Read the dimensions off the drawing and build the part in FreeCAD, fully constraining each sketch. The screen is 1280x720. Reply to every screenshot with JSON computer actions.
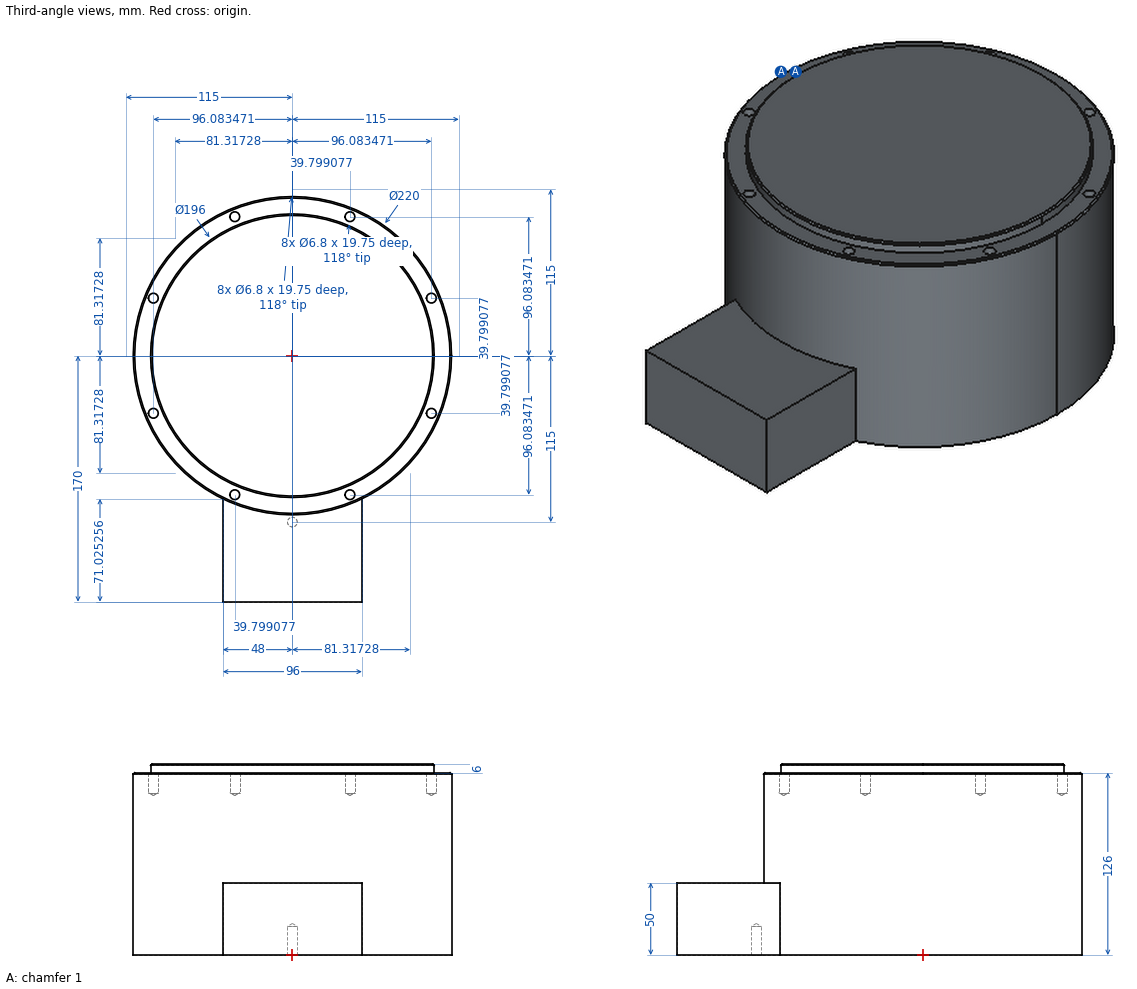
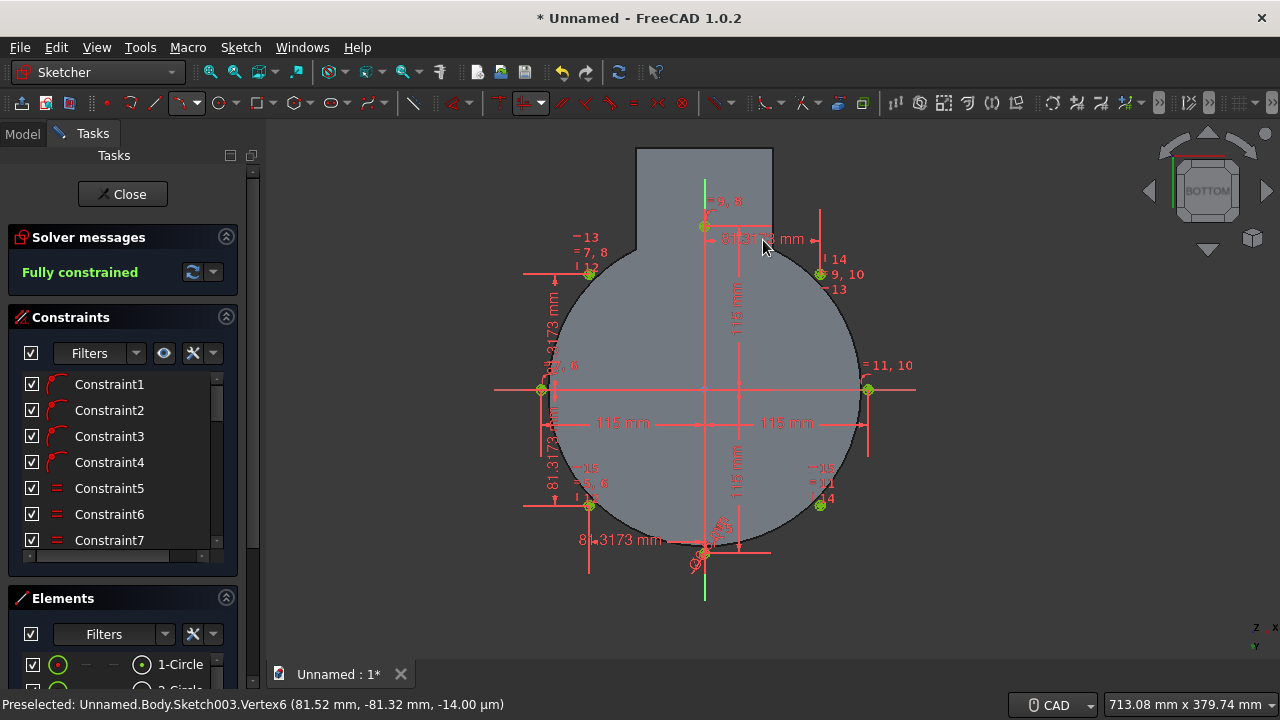
{"action": "left_click", "coordinate": [123, 194]}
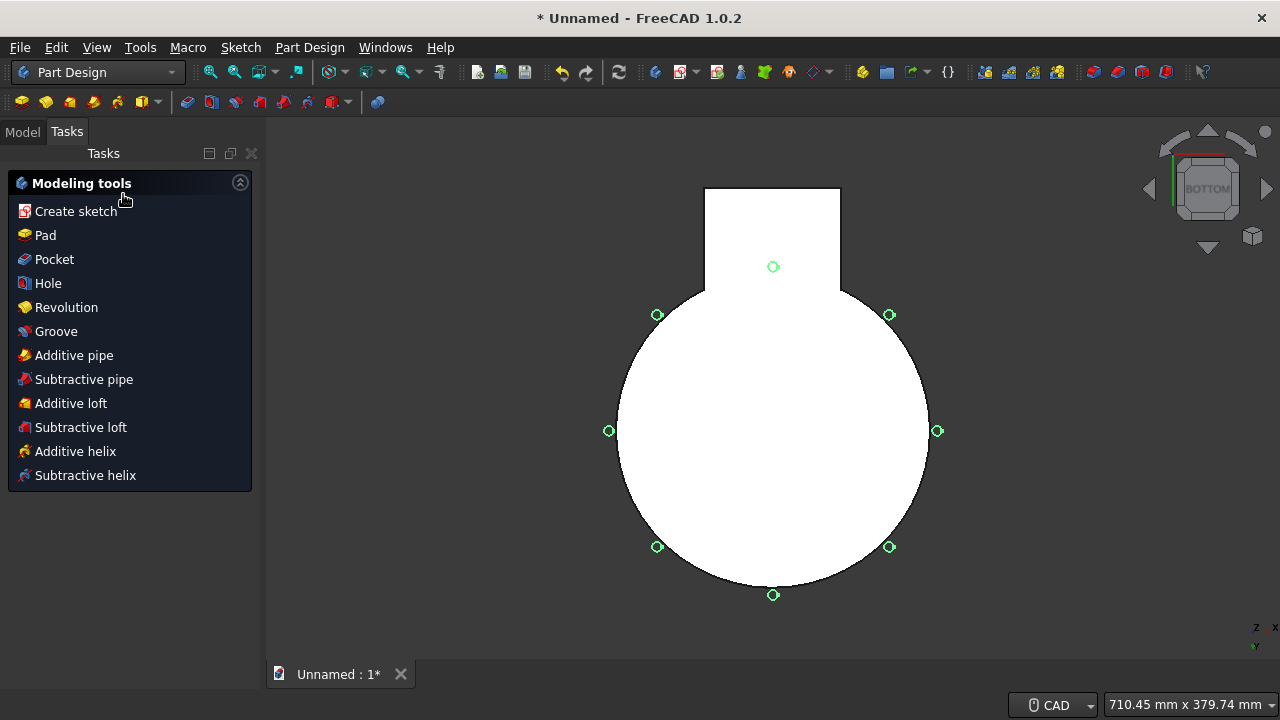
{"action": "left_click", "coordinate": [212, 102]}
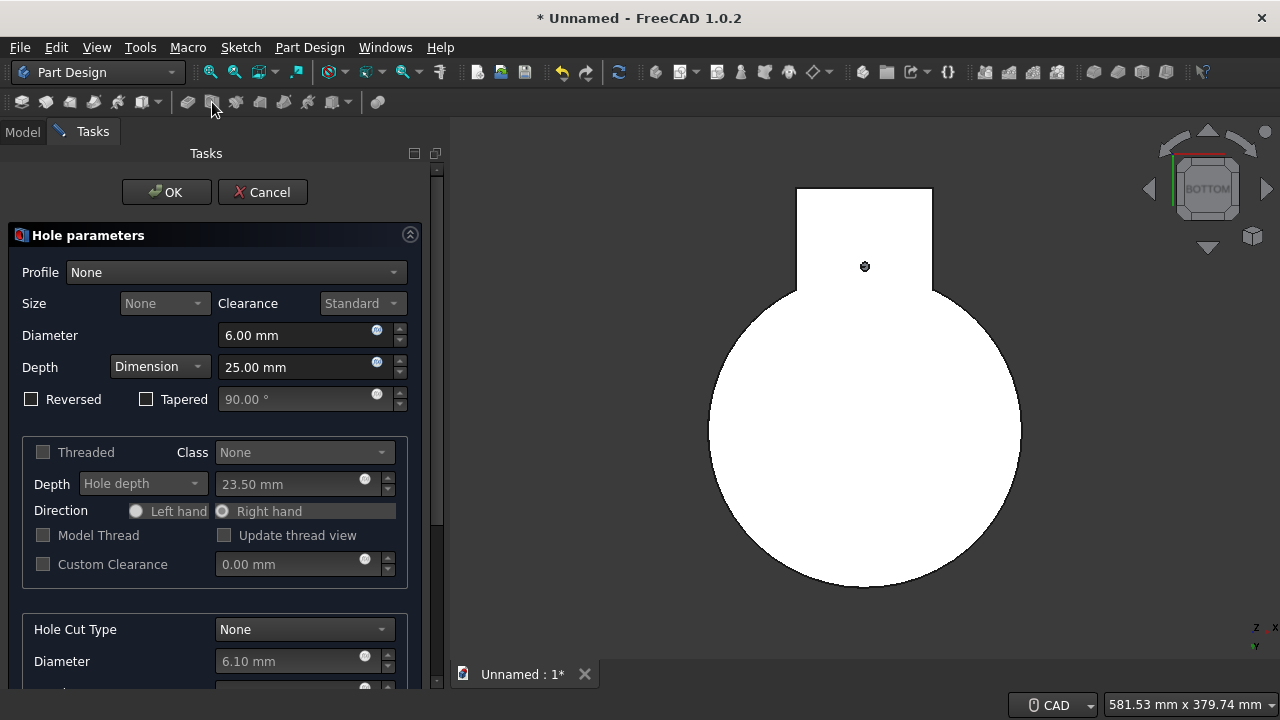
{"action": "triple_click", "coordinate": [305, 335]}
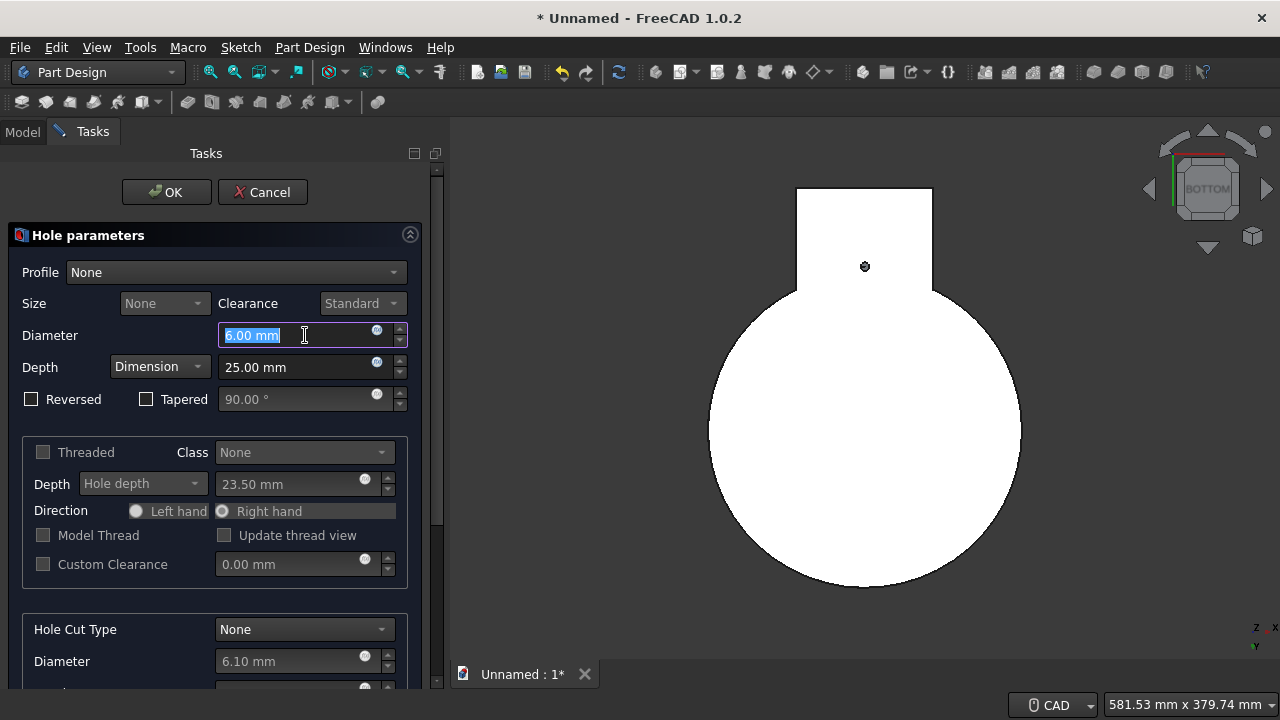
{"action": "type", "text": "6.8"}
{"action": "key", "text": "Tab"}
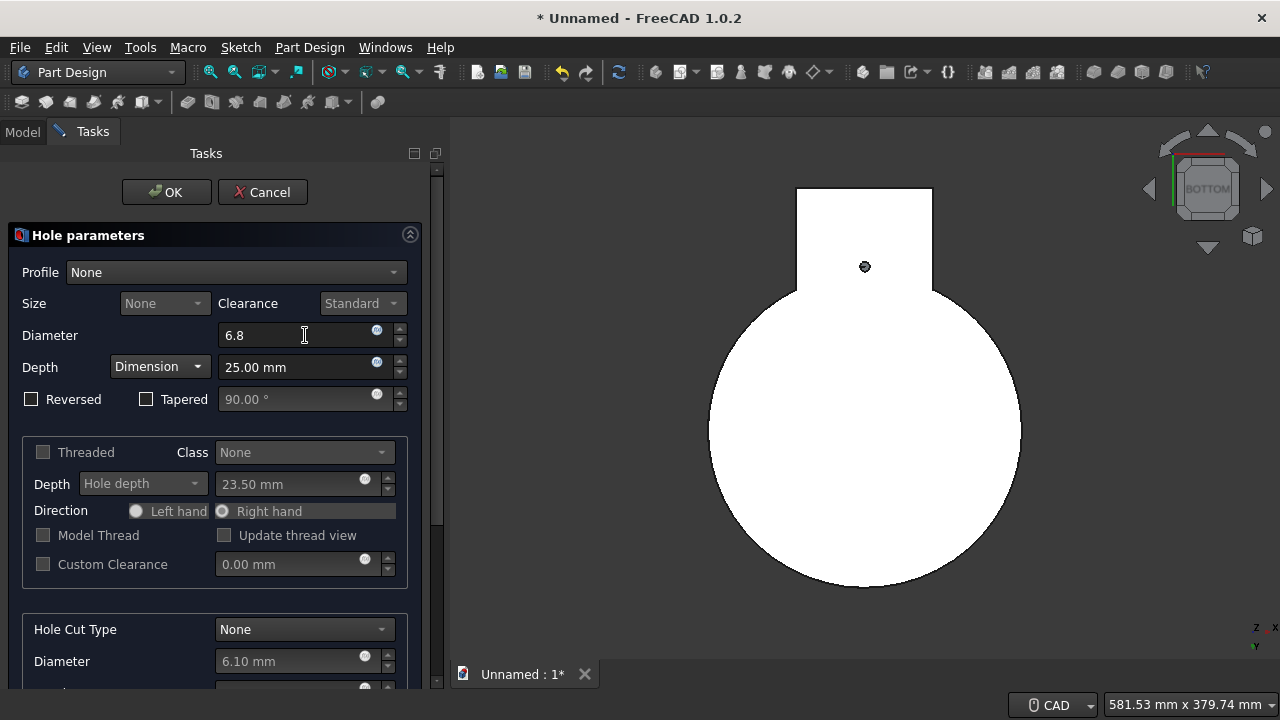
{"action": "triple_click", "coordinate": [305, 367]}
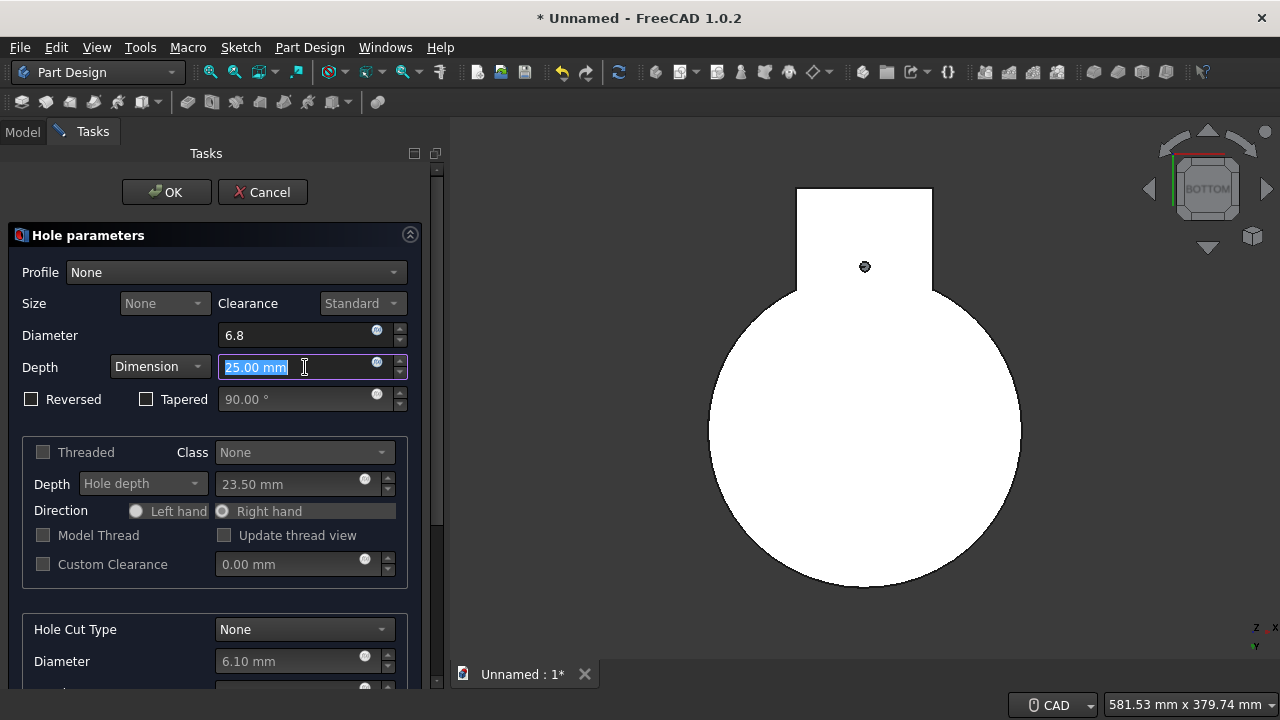
{"action": "type", "text": "19.75"}
{"action": "key", "text": "Tab"}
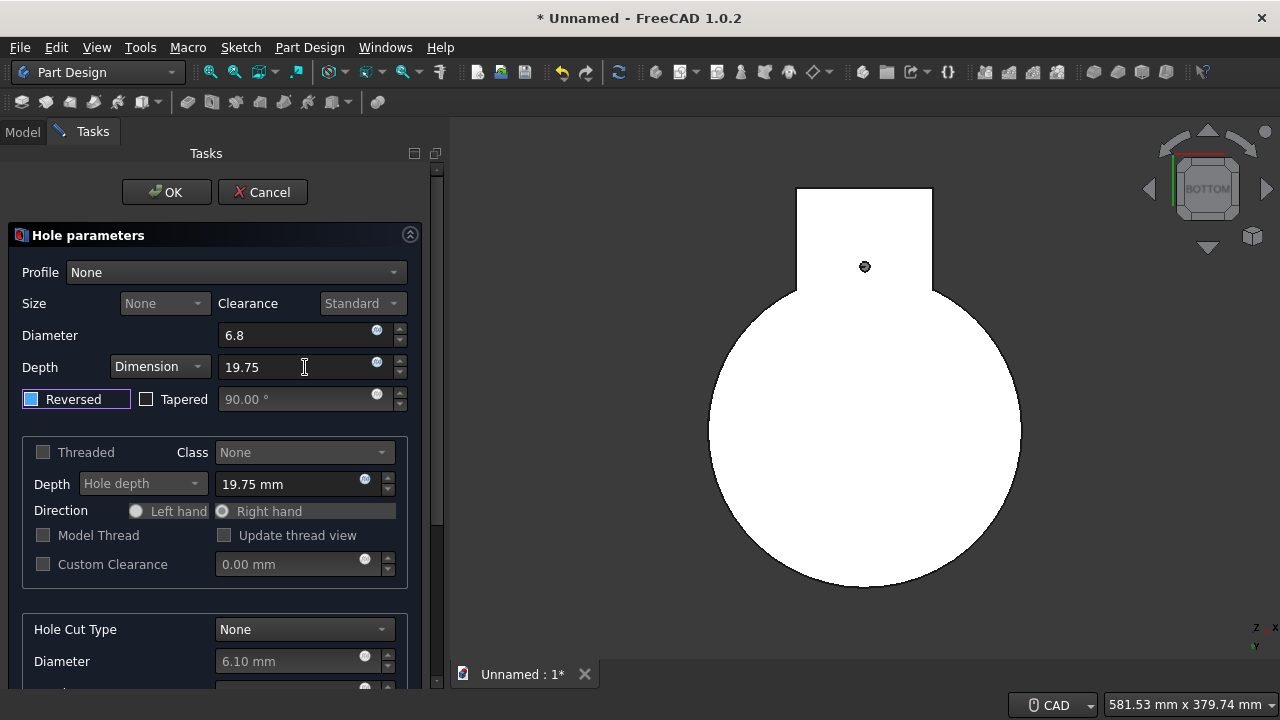
{"action": "left_click", "coordinate": [167, 192]}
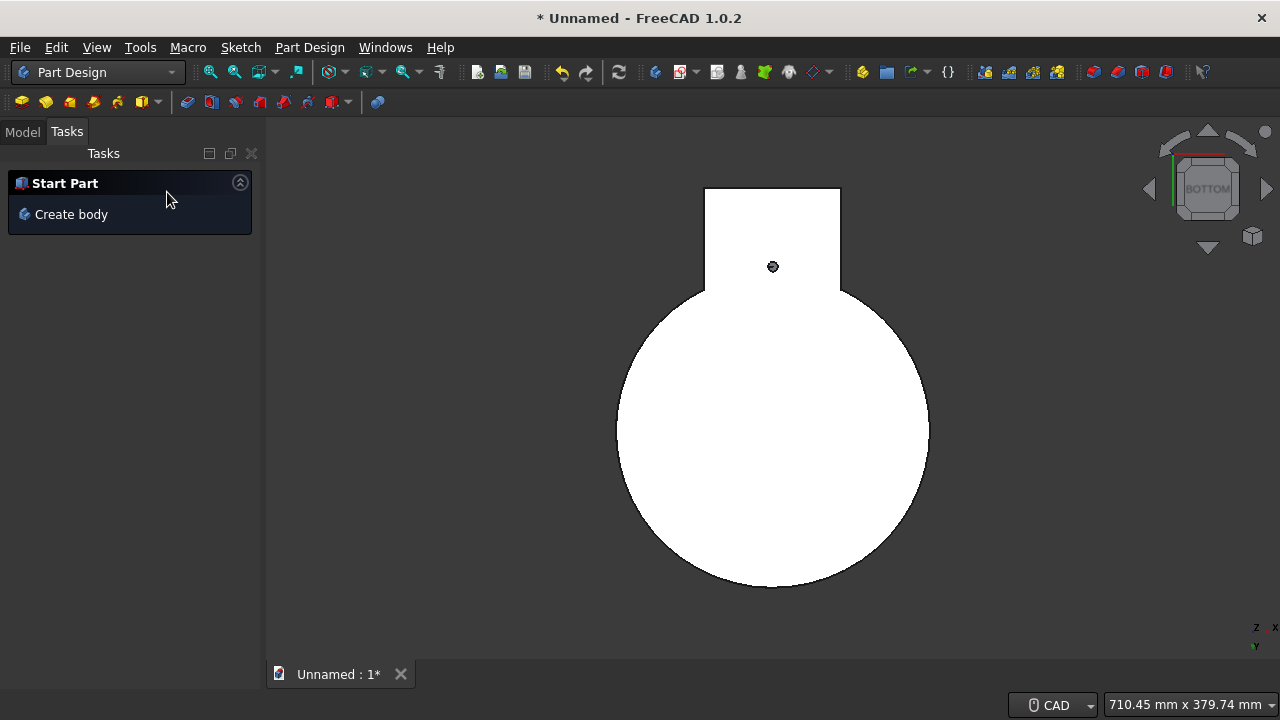
{"action": "key", "text": "0"}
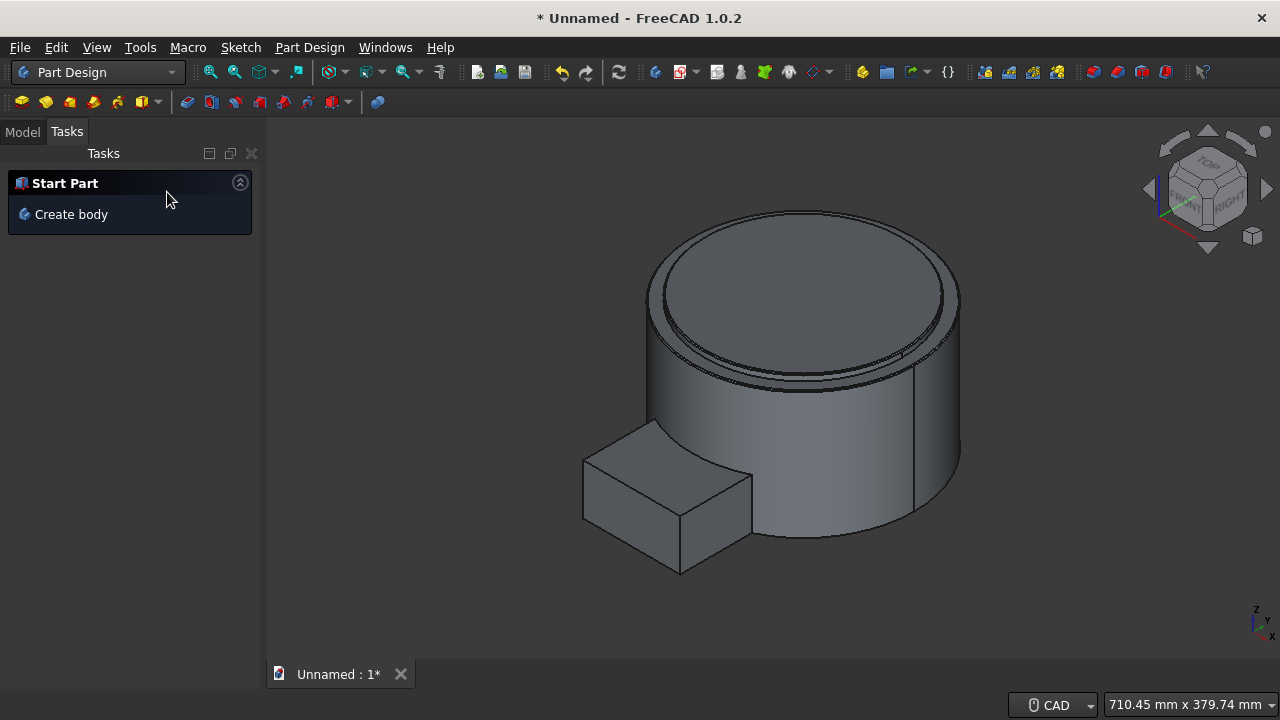
{"action": "left_click", "coordinate": [803, 293]}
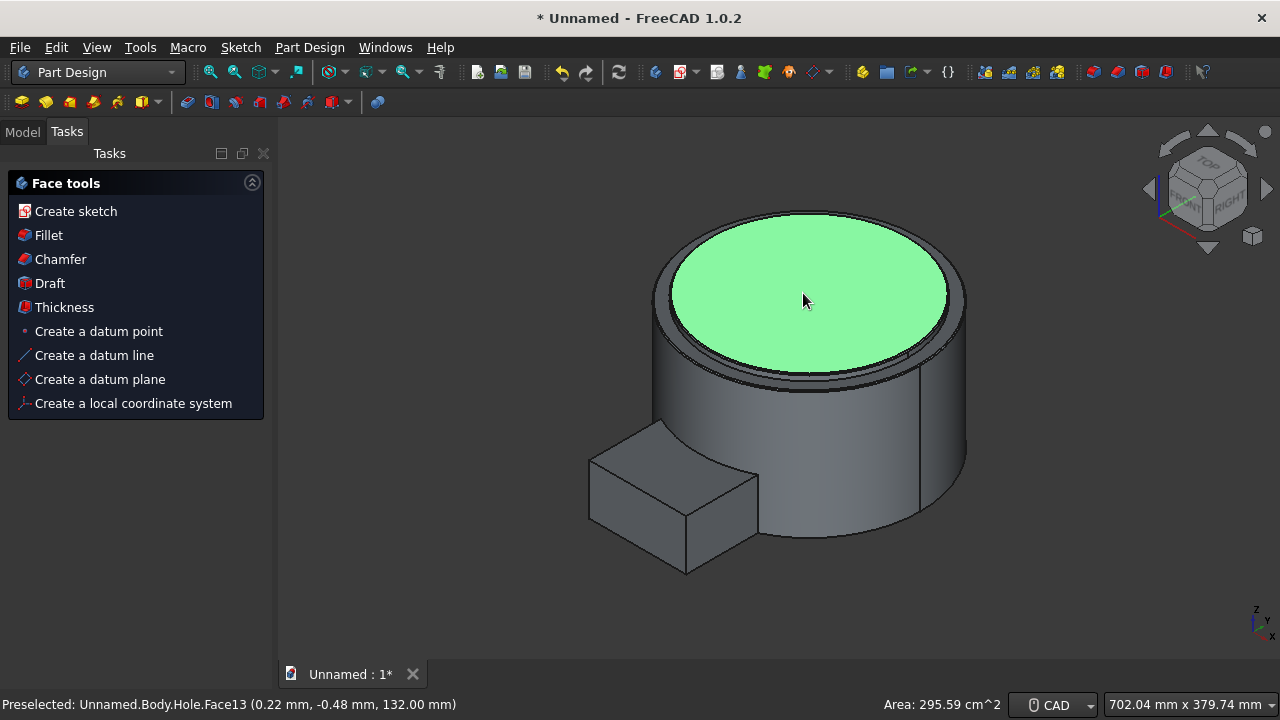
{"action": "left_click", "coordinate": [680, 72]}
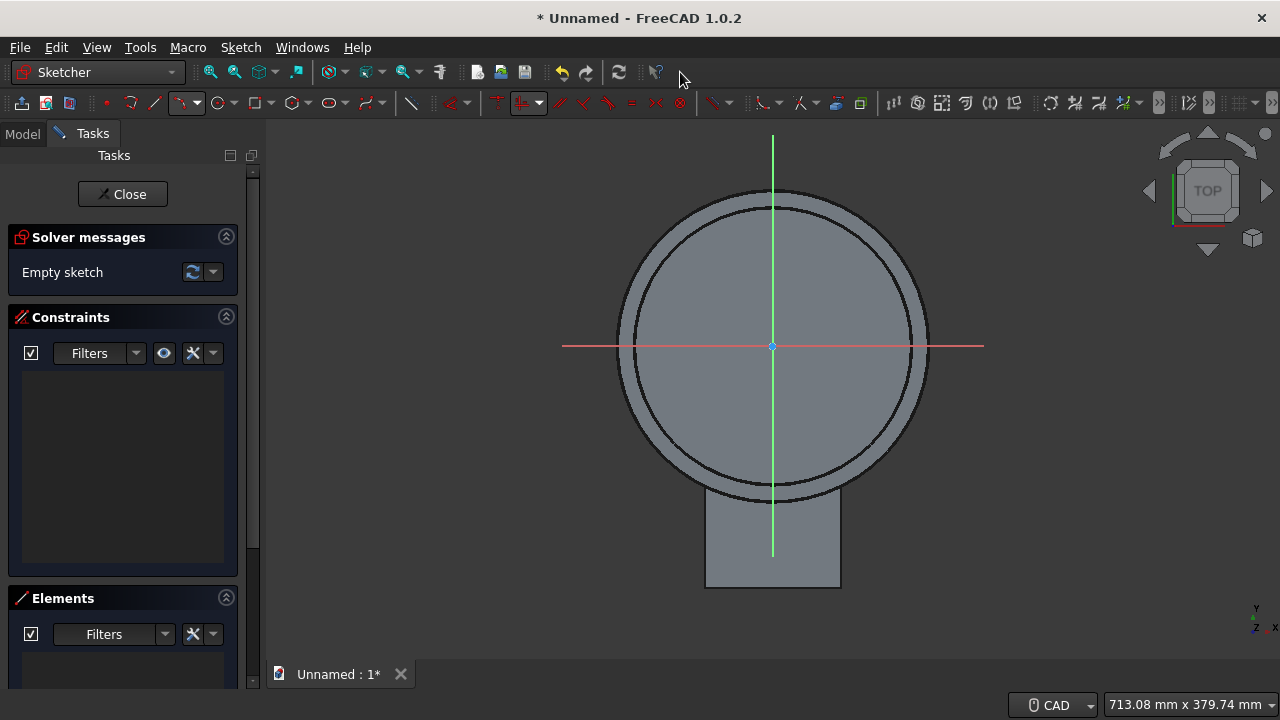
{"action": "left_click", "coordinate": [218, 104]}